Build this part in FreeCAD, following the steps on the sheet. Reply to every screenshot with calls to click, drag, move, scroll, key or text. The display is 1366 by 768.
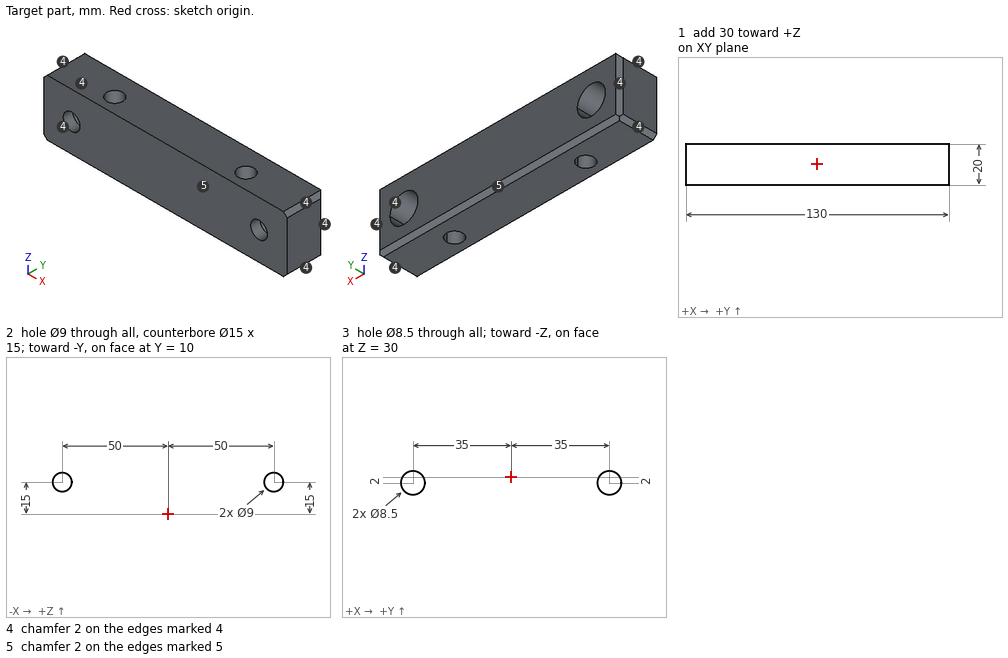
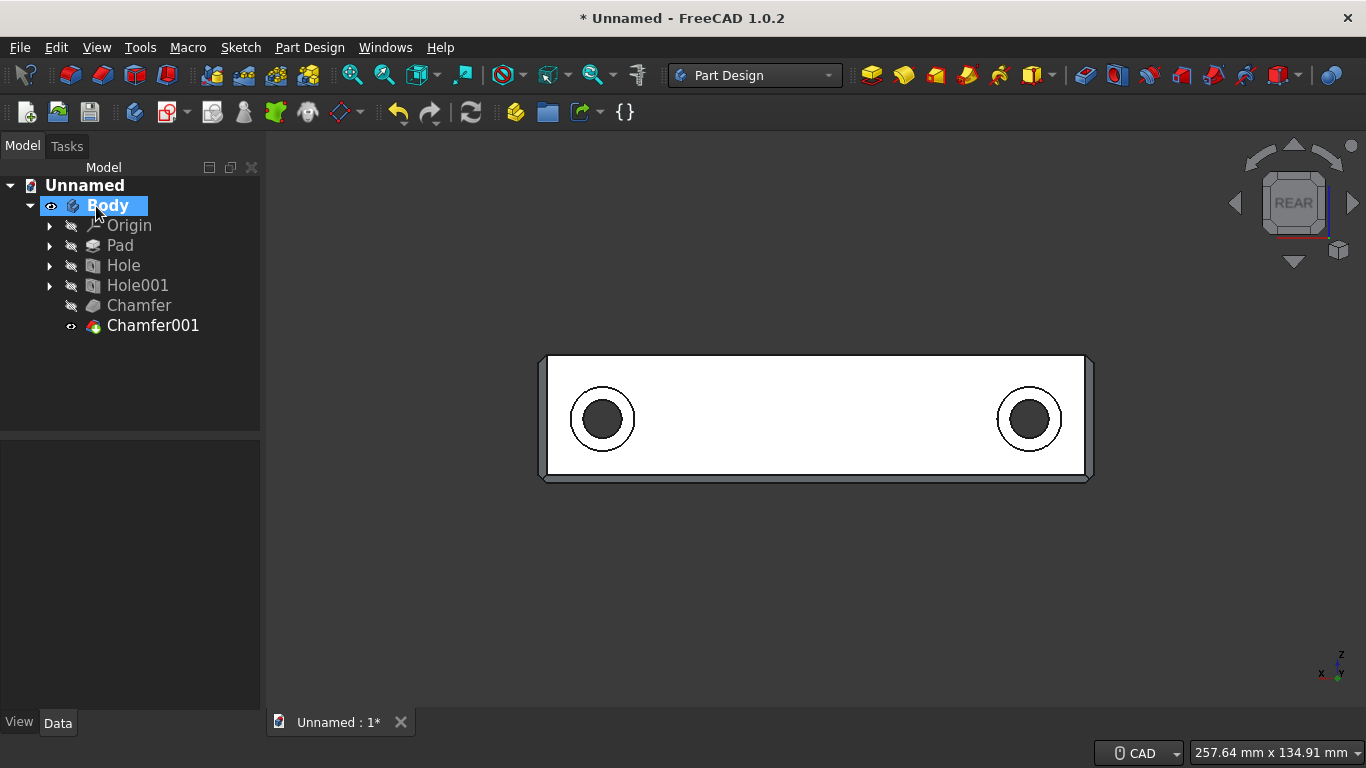
key(0)